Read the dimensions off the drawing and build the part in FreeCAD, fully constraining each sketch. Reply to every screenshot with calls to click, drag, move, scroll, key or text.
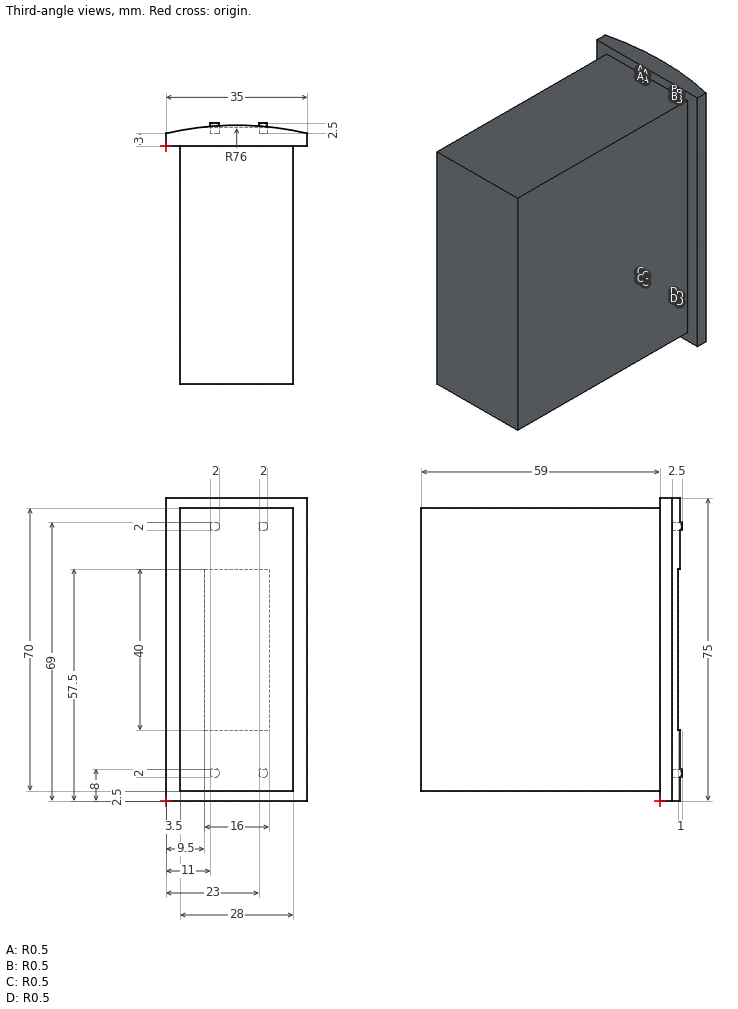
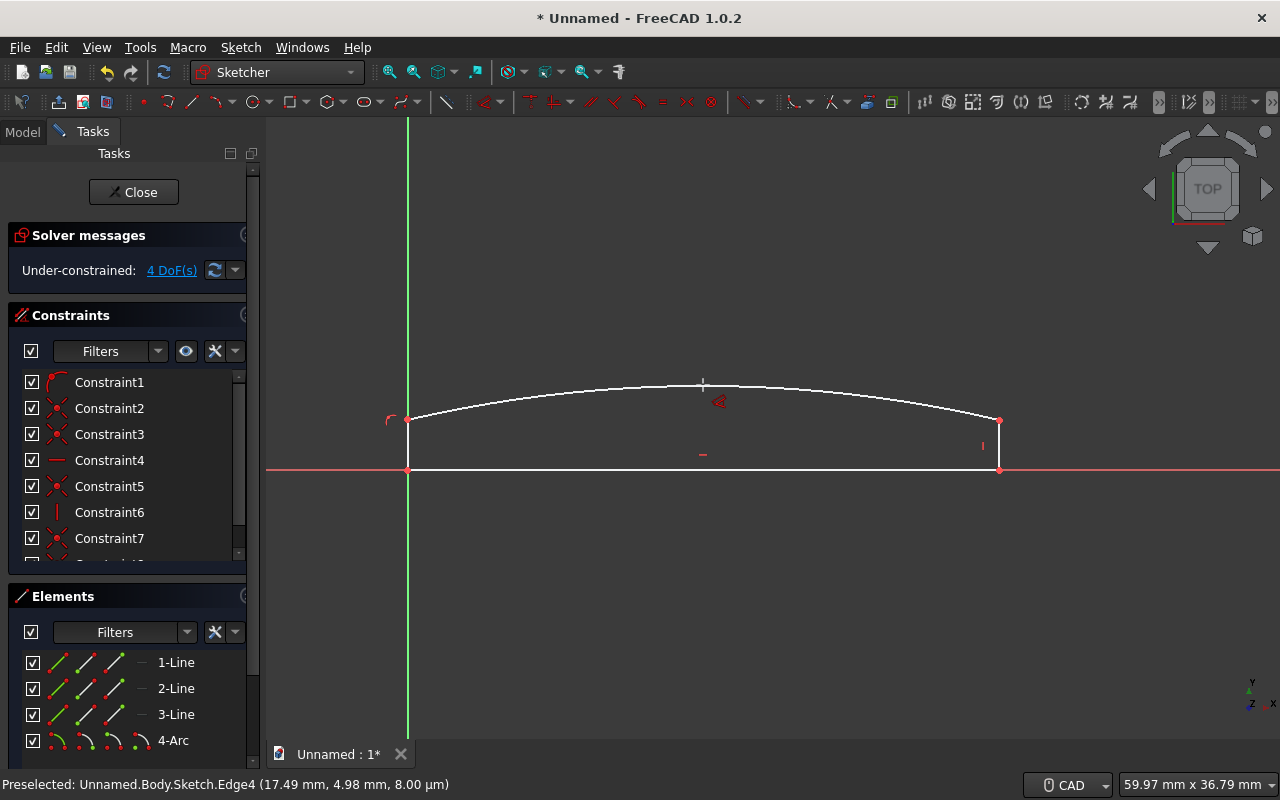
click(822, 391)
click(825, 359)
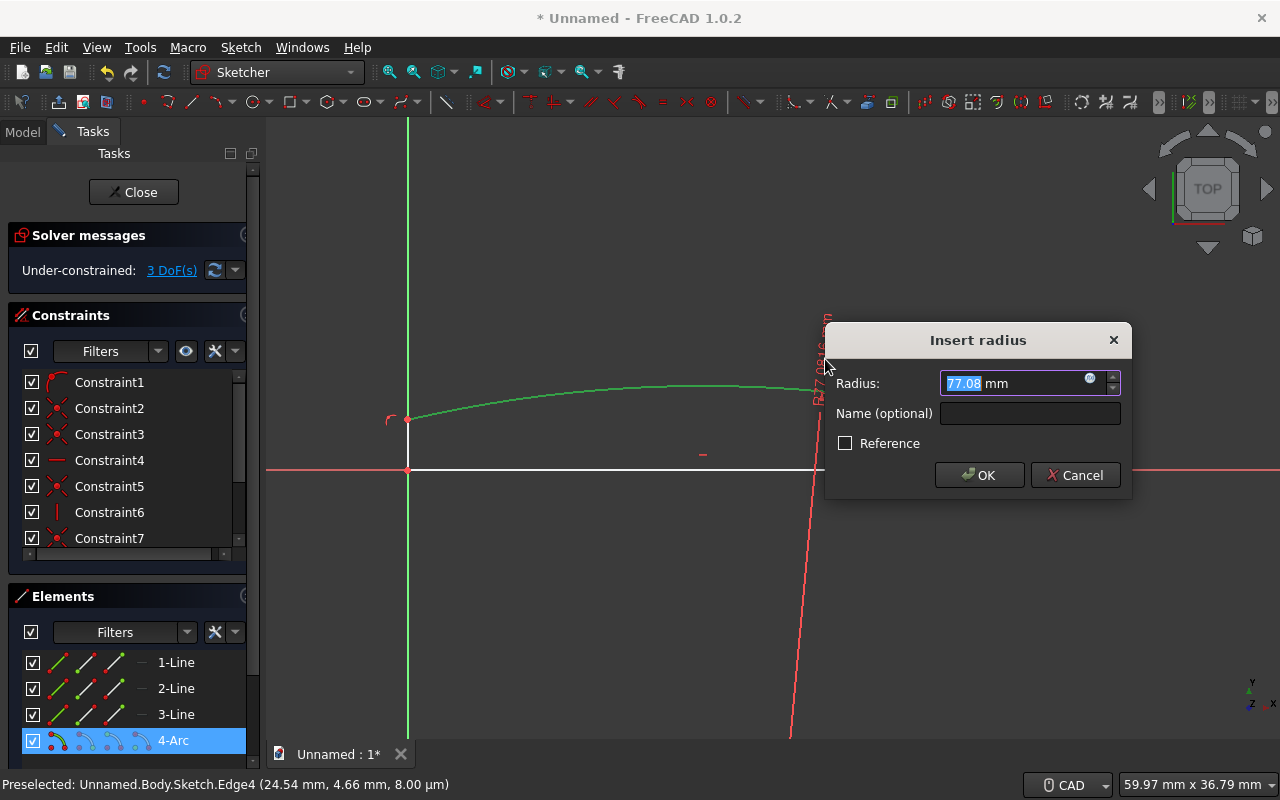
text(76)
key(Return)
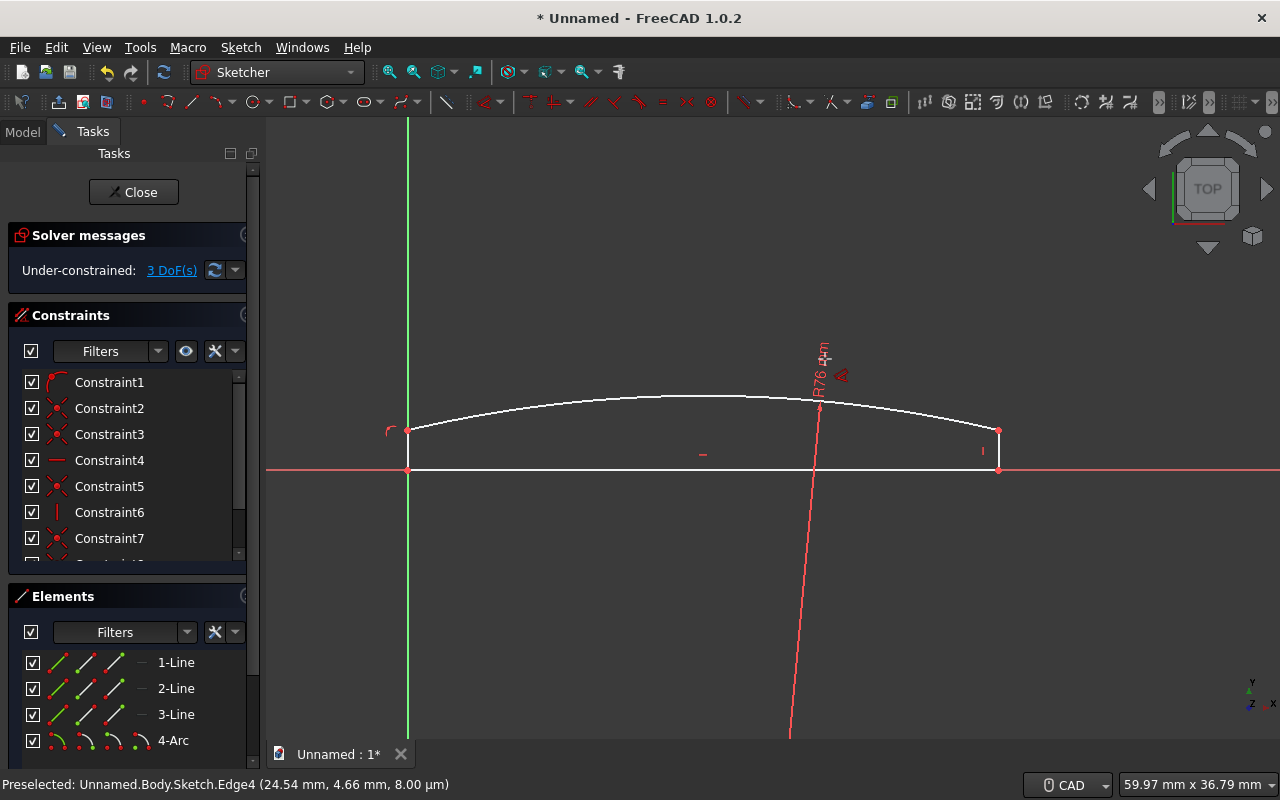
click(408, 442)
click(374, 450)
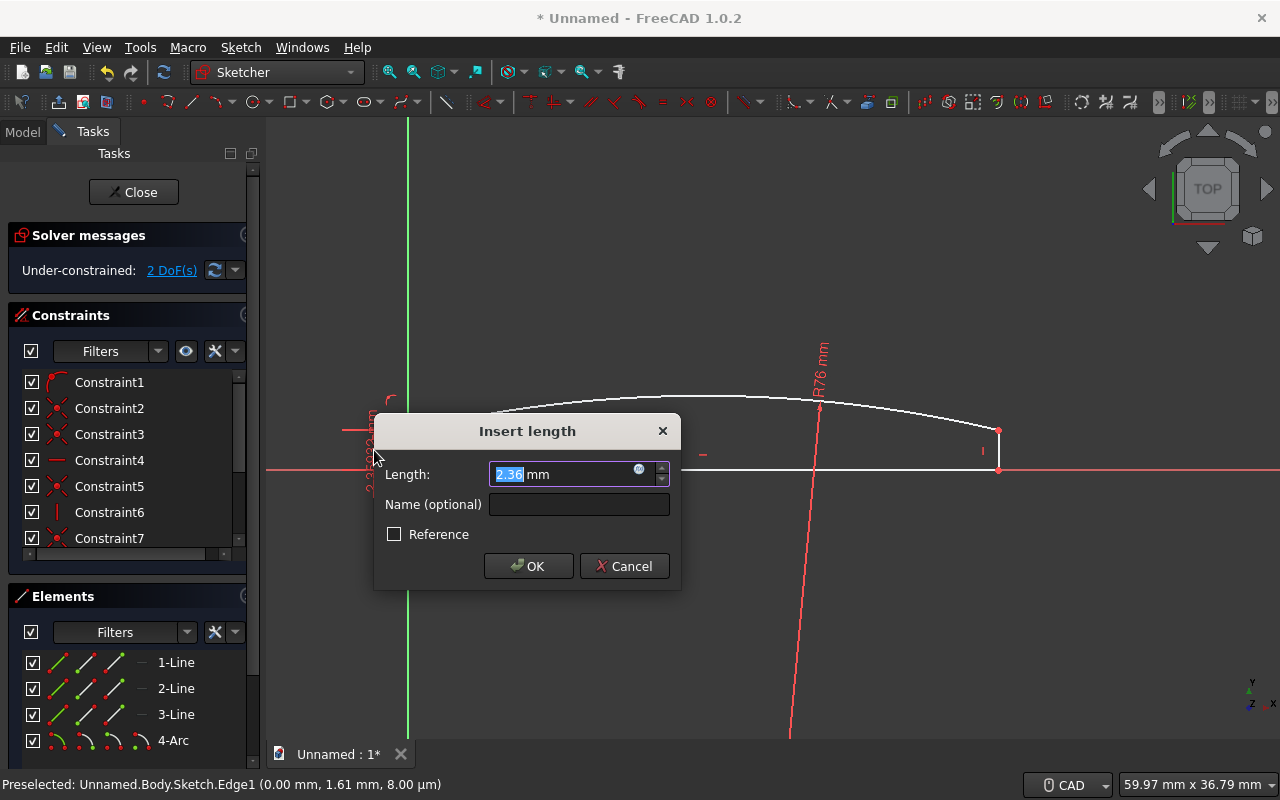
text(3)
key(Return)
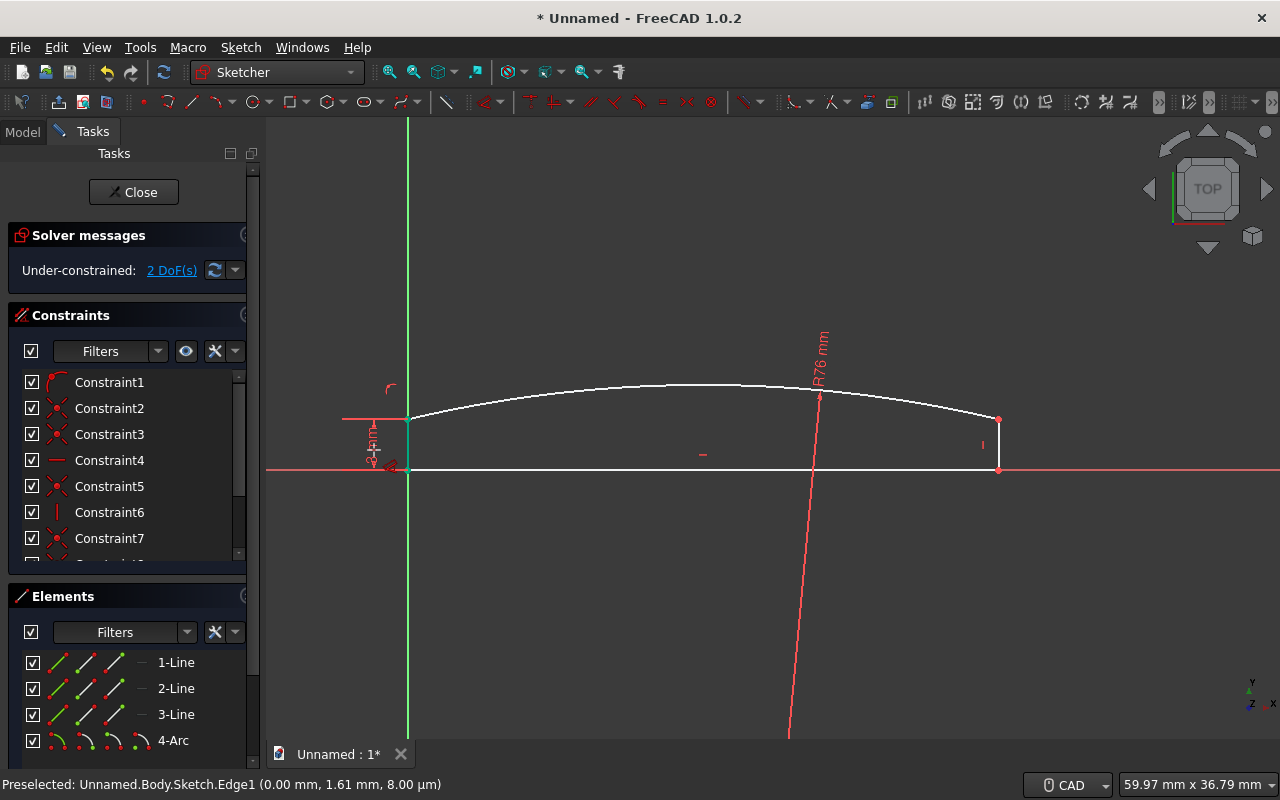
click(999, 455)
click(1033, 445)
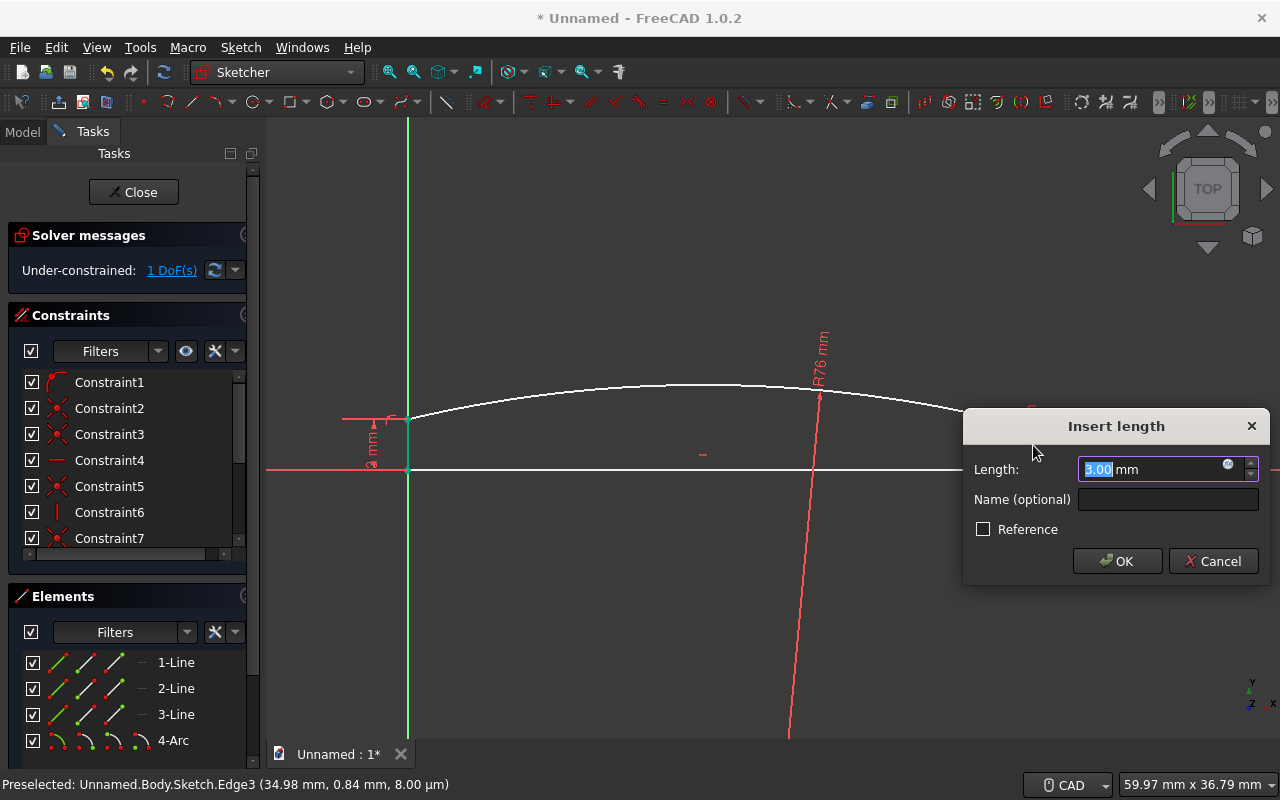
text(3)
key(Return)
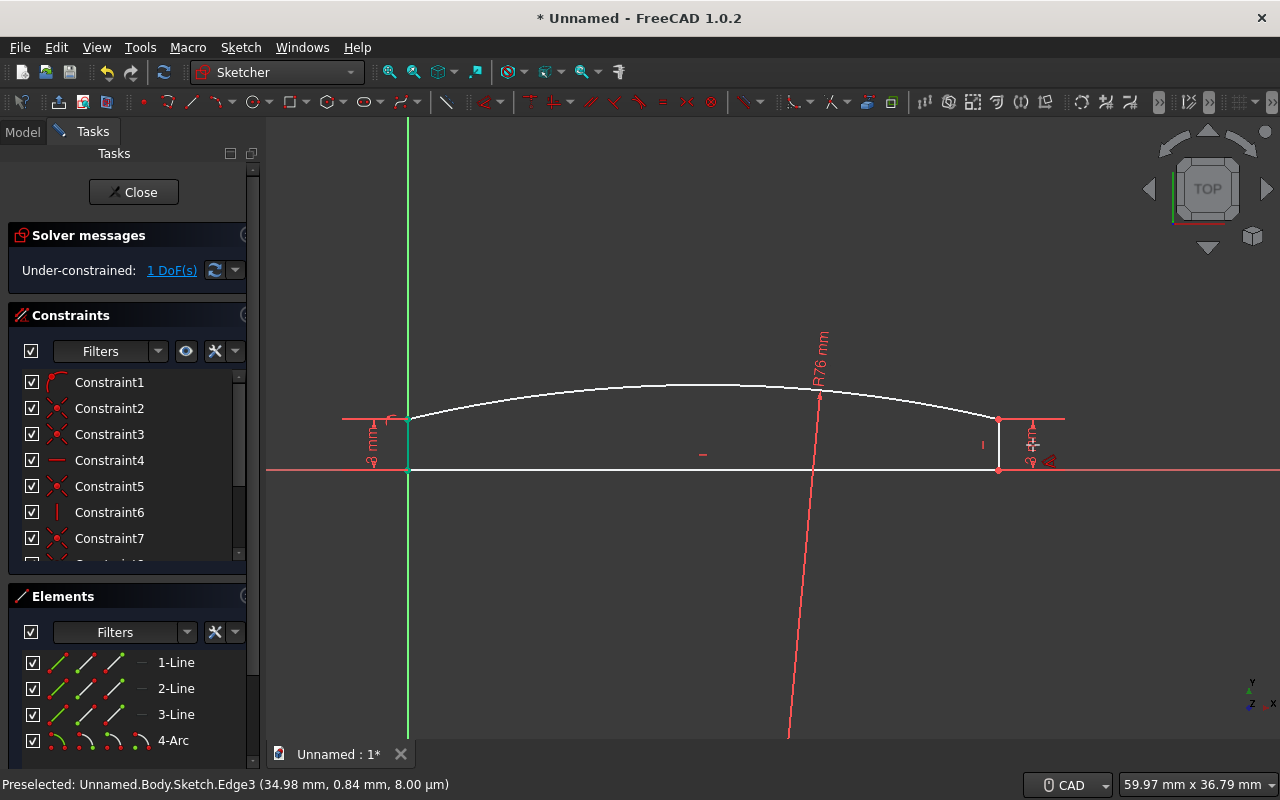
click(585, 470)
click(703, 504)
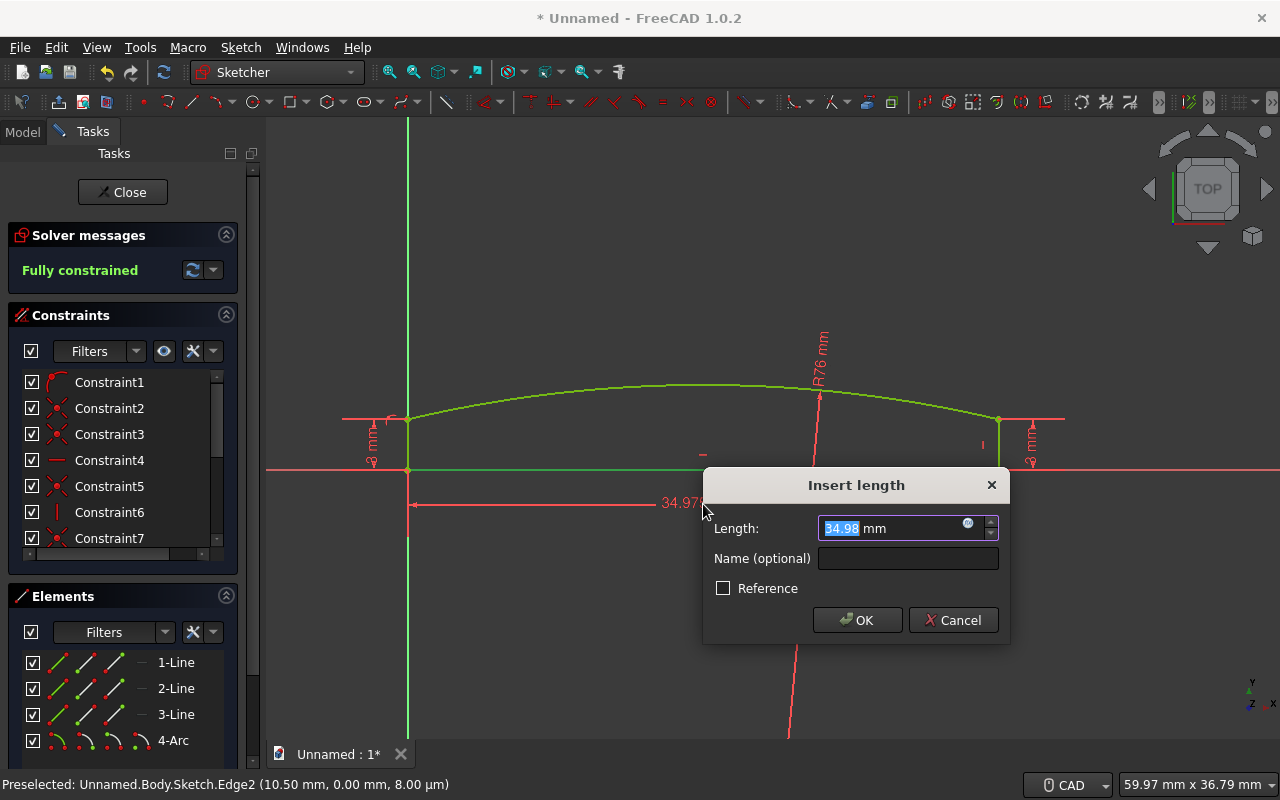
text(35)
key(Return)
key(Escape)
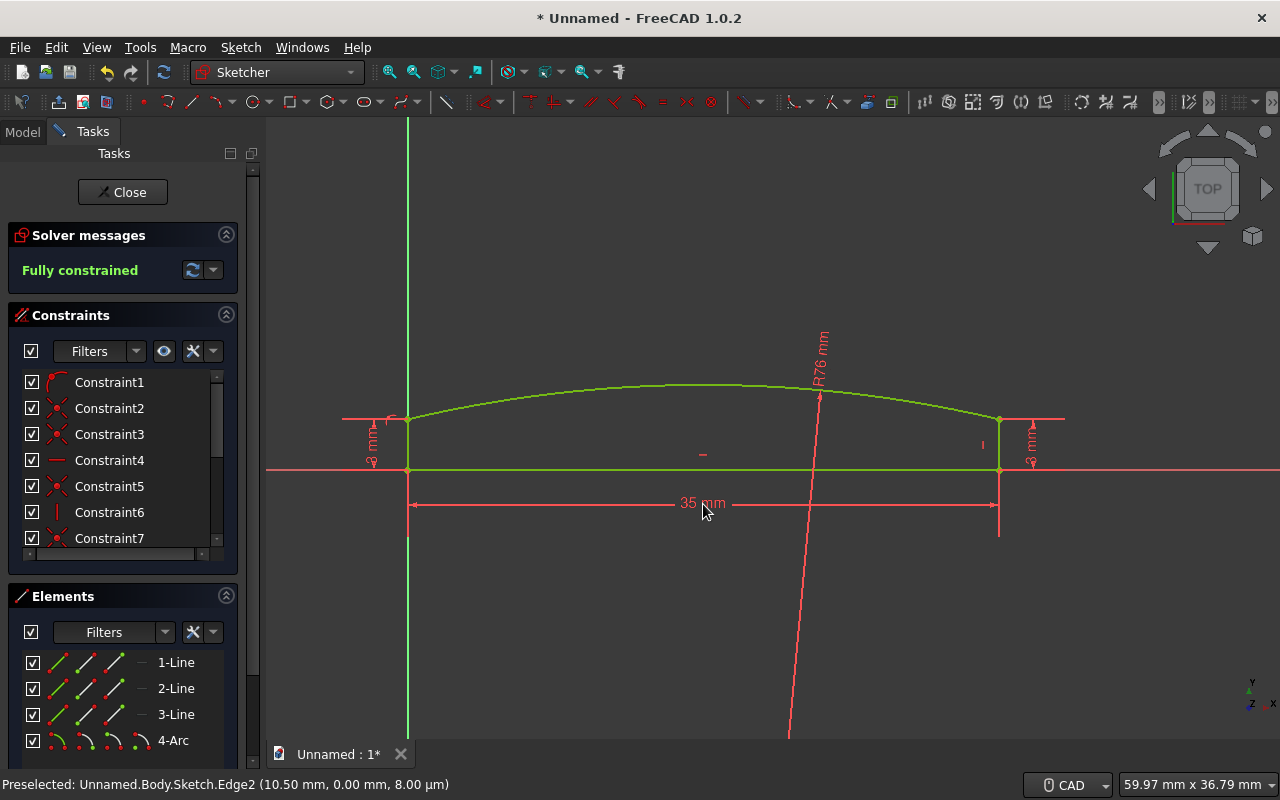
click(123, 192)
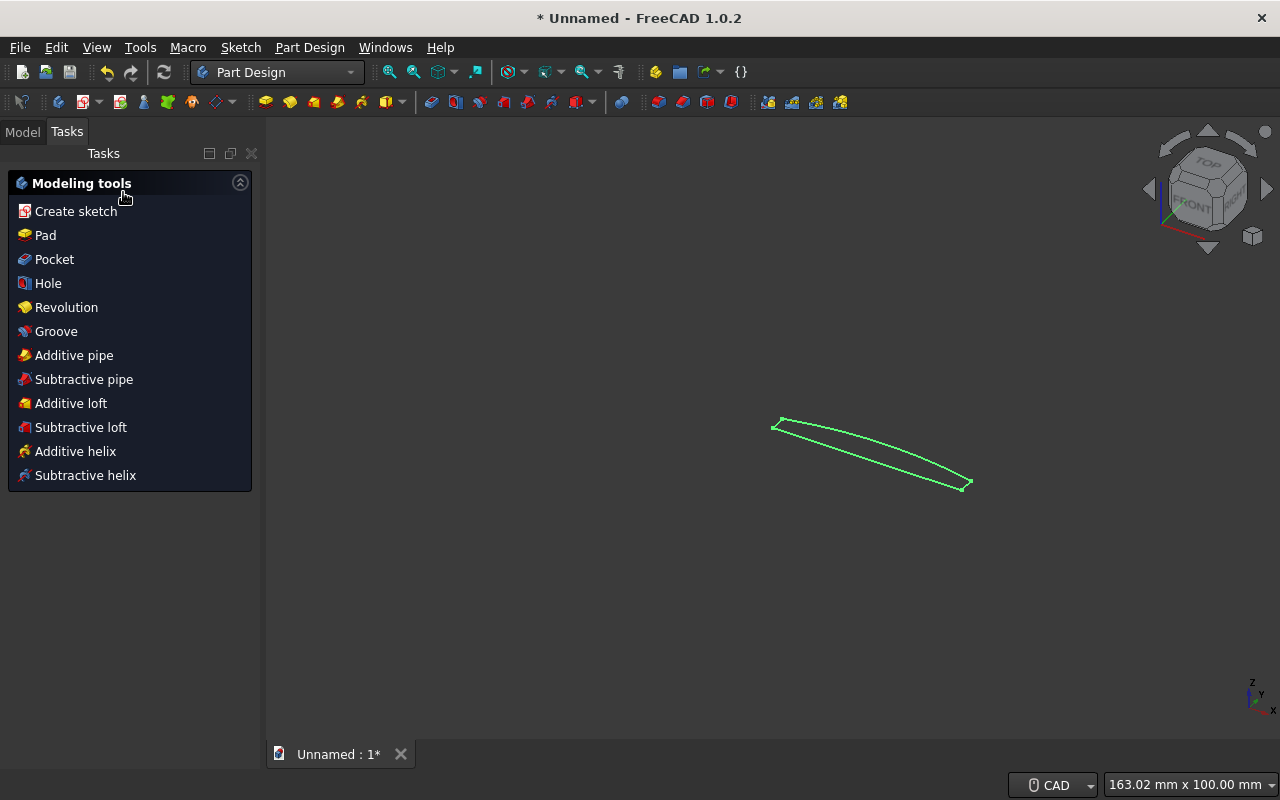
click(266, 102)